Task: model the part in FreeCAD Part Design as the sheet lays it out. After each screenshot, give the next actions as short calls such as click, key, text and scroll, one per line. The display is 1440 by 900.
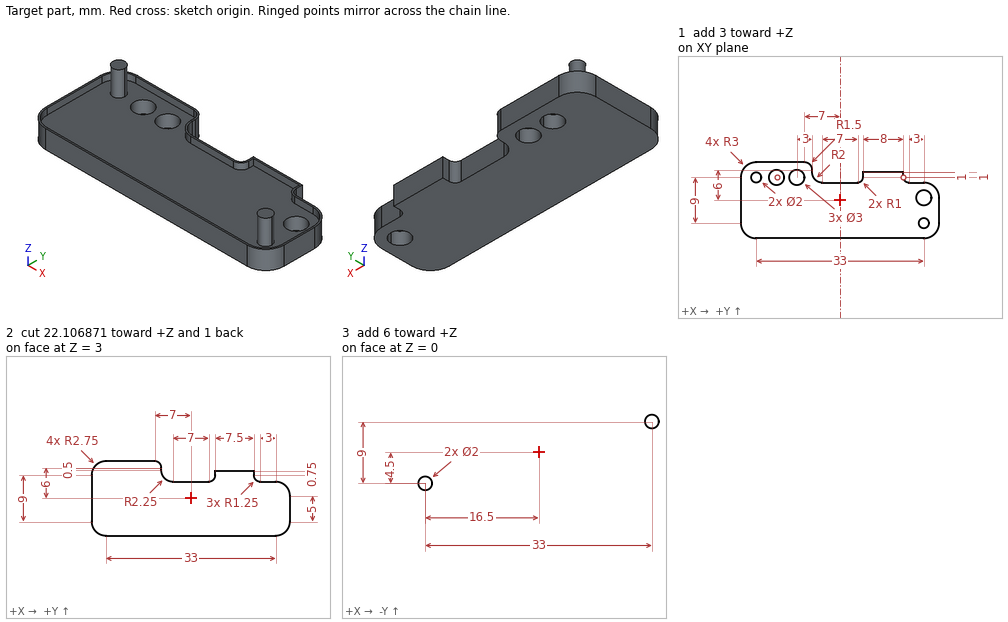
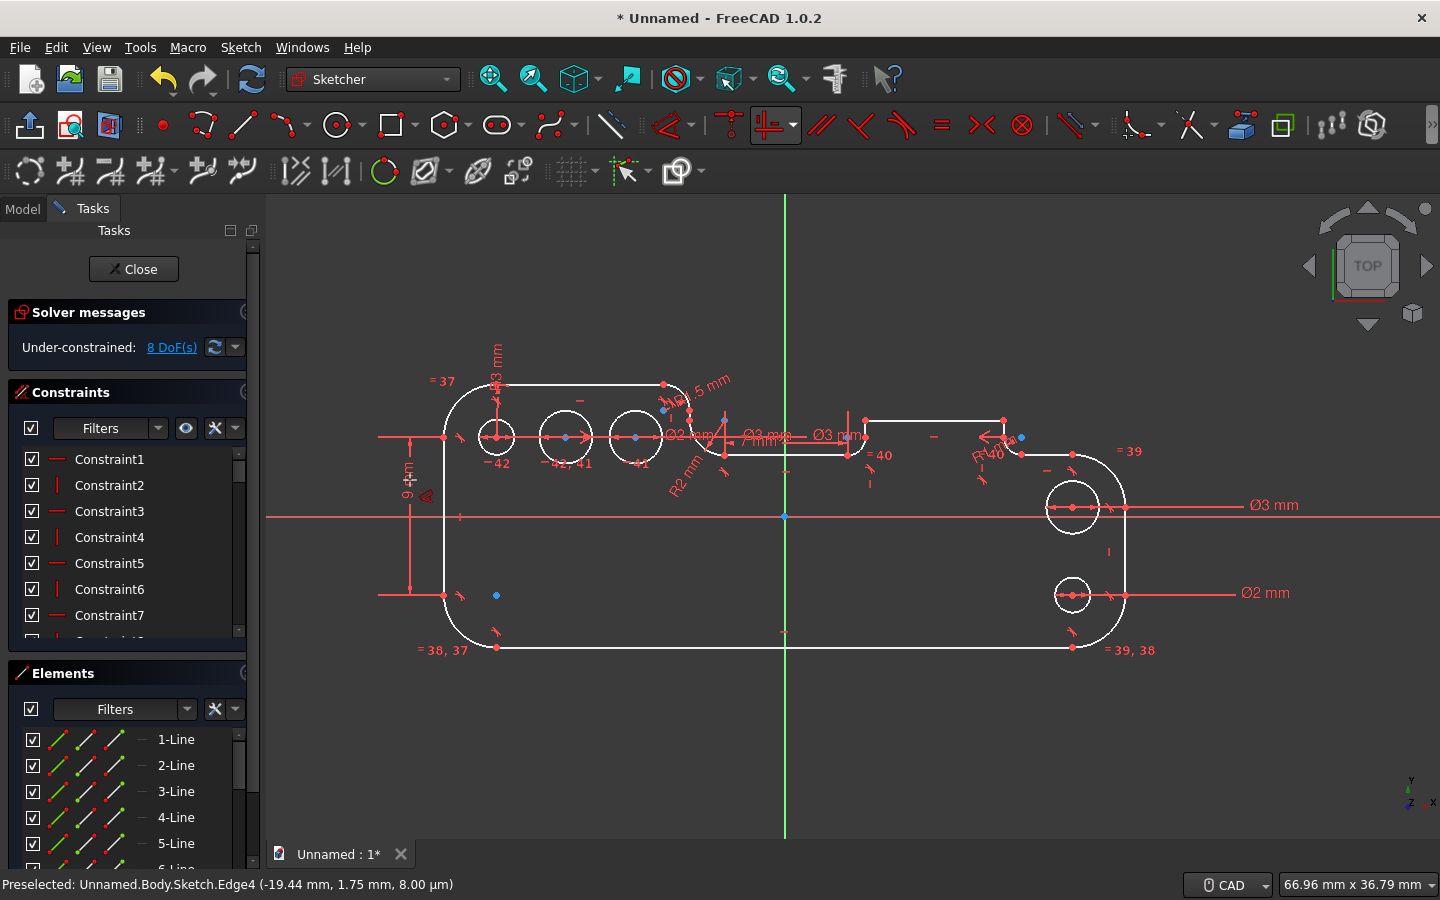
click(1057, 455)
click(1047, 421)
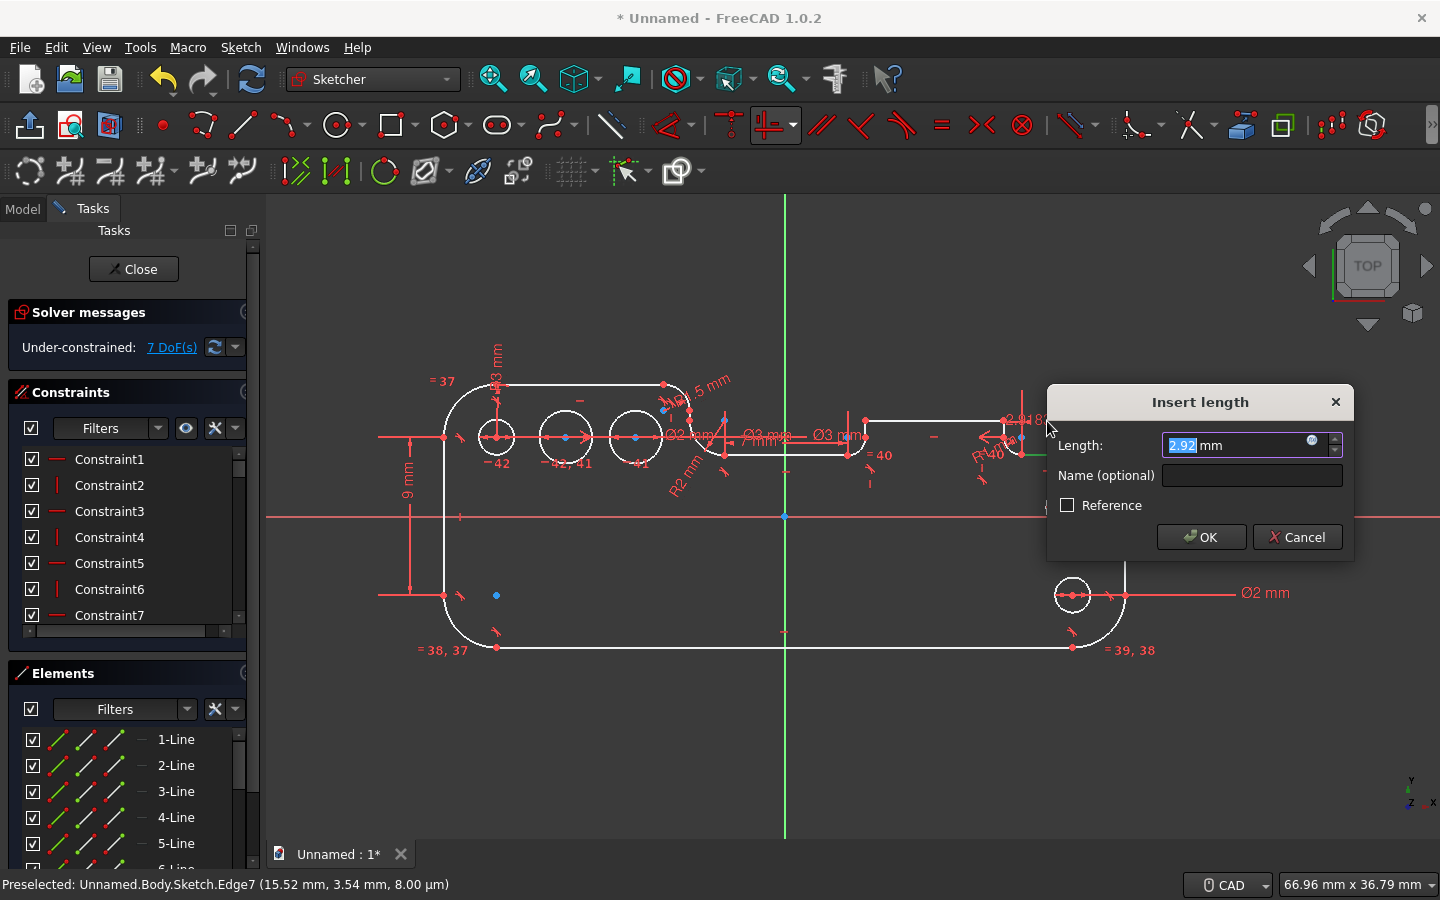
text(3)
key(Return)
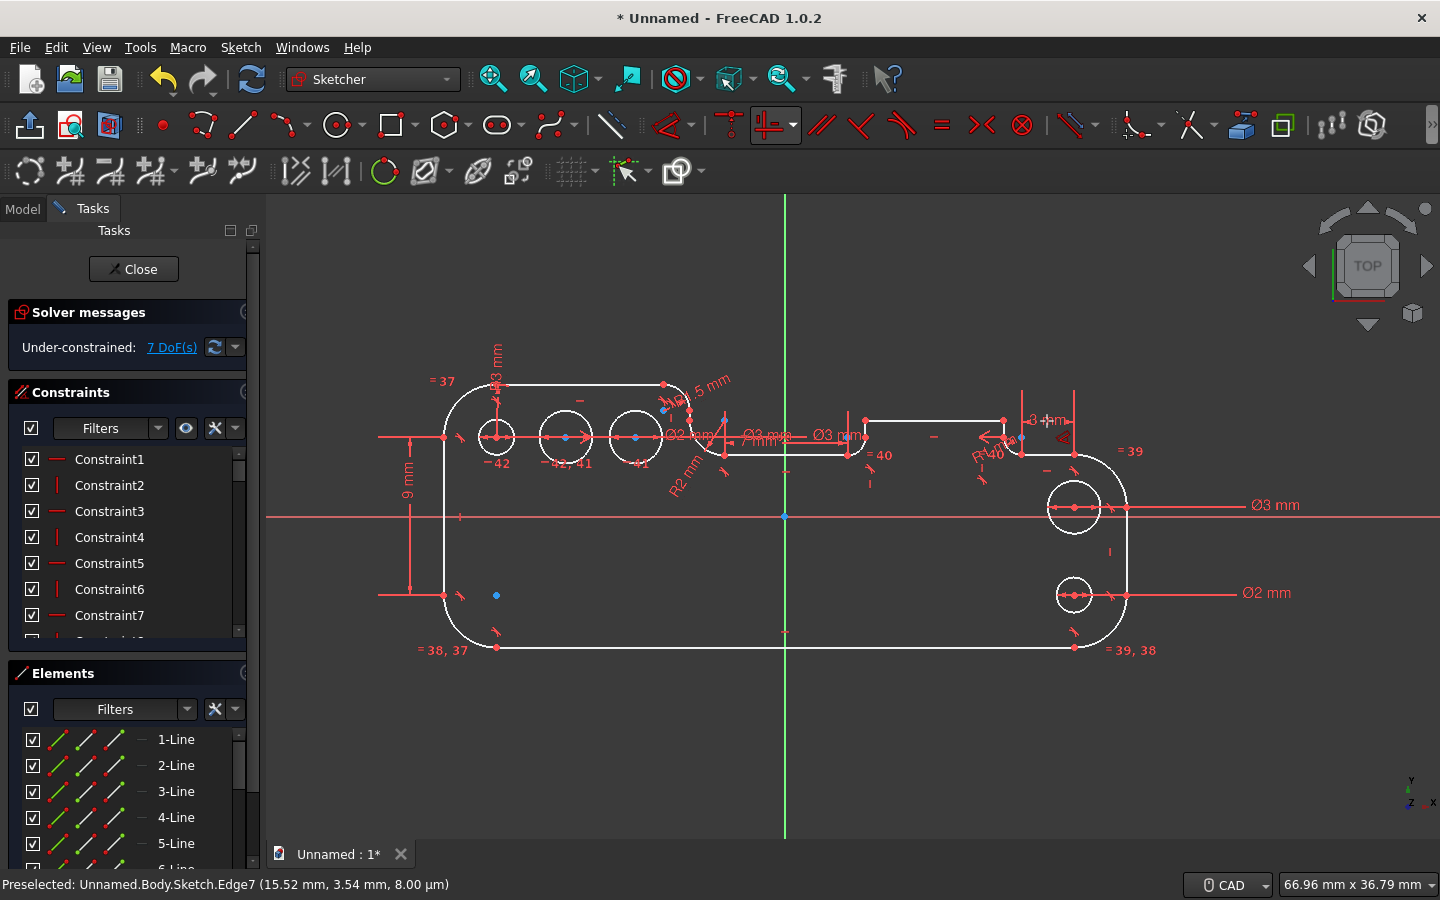
scroll(1004, 429, up, 5)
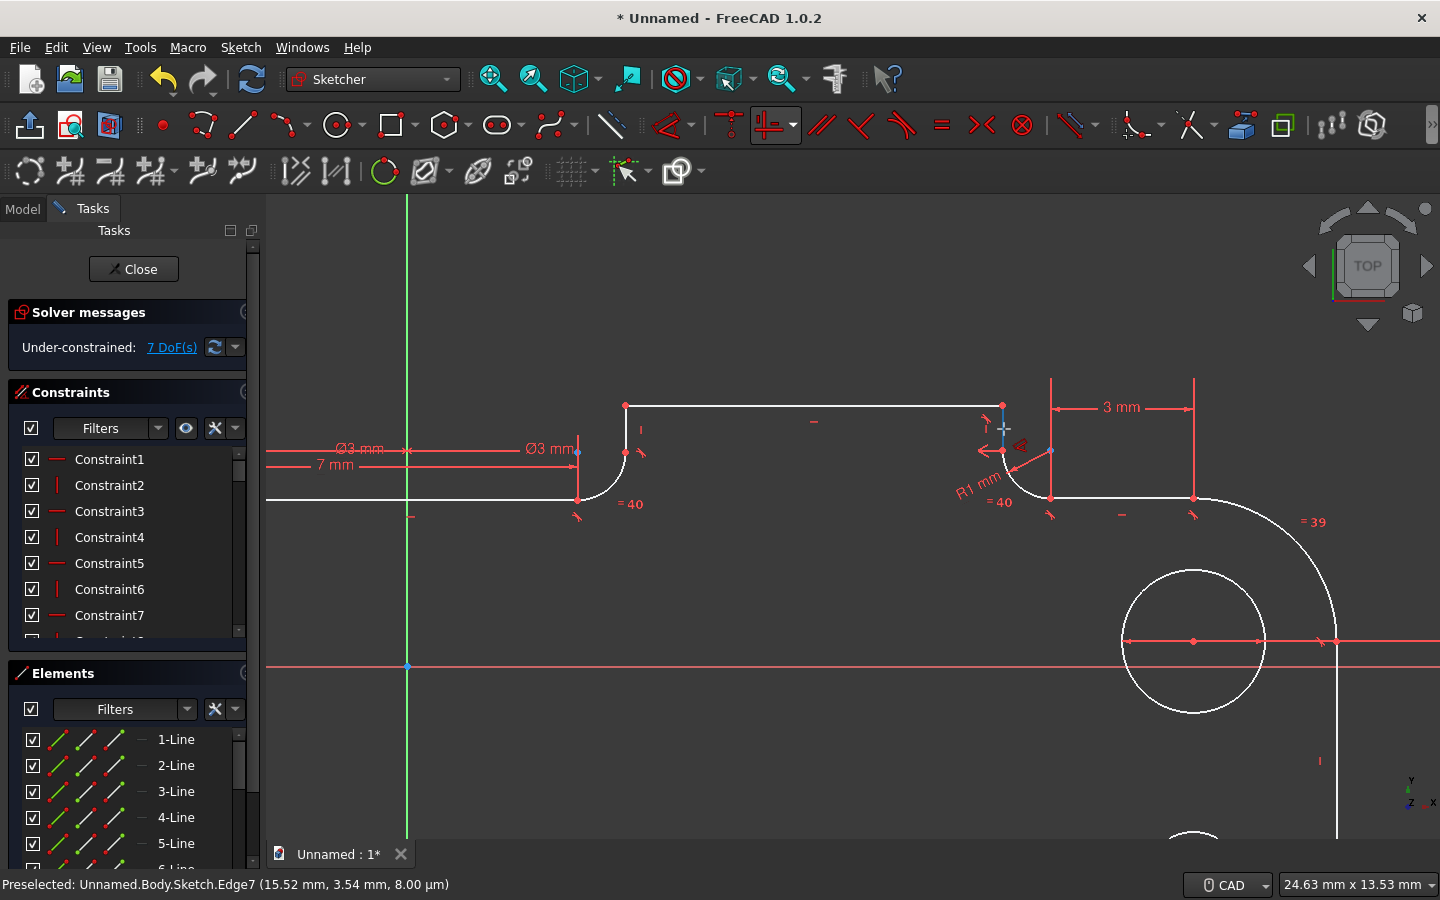
click(1003, 428)
click(1037, 428)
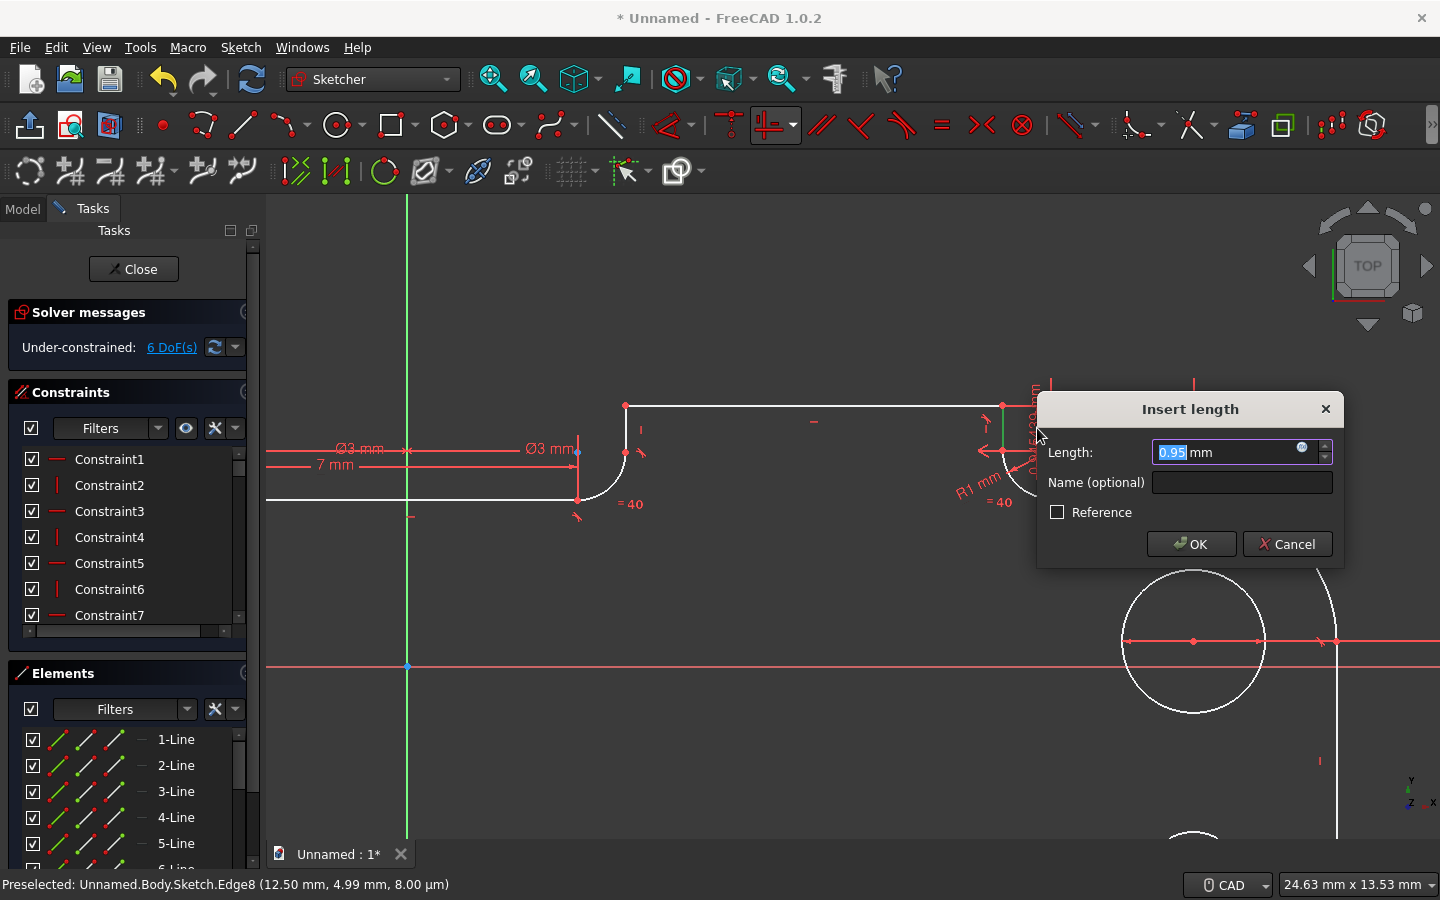
text(1)
key(Return)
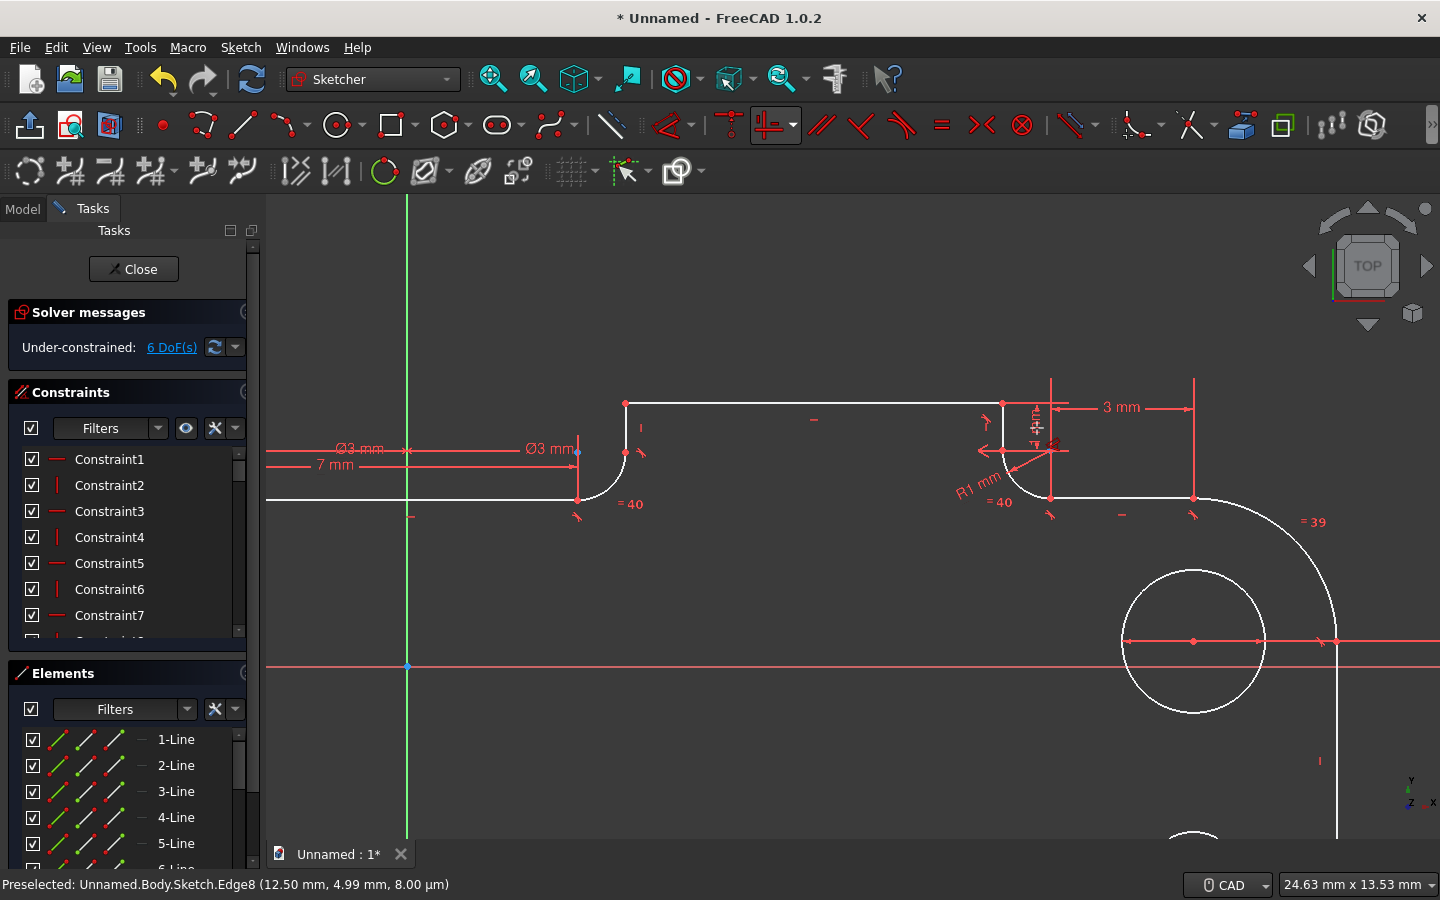
click(890, 403)
click(814, 369)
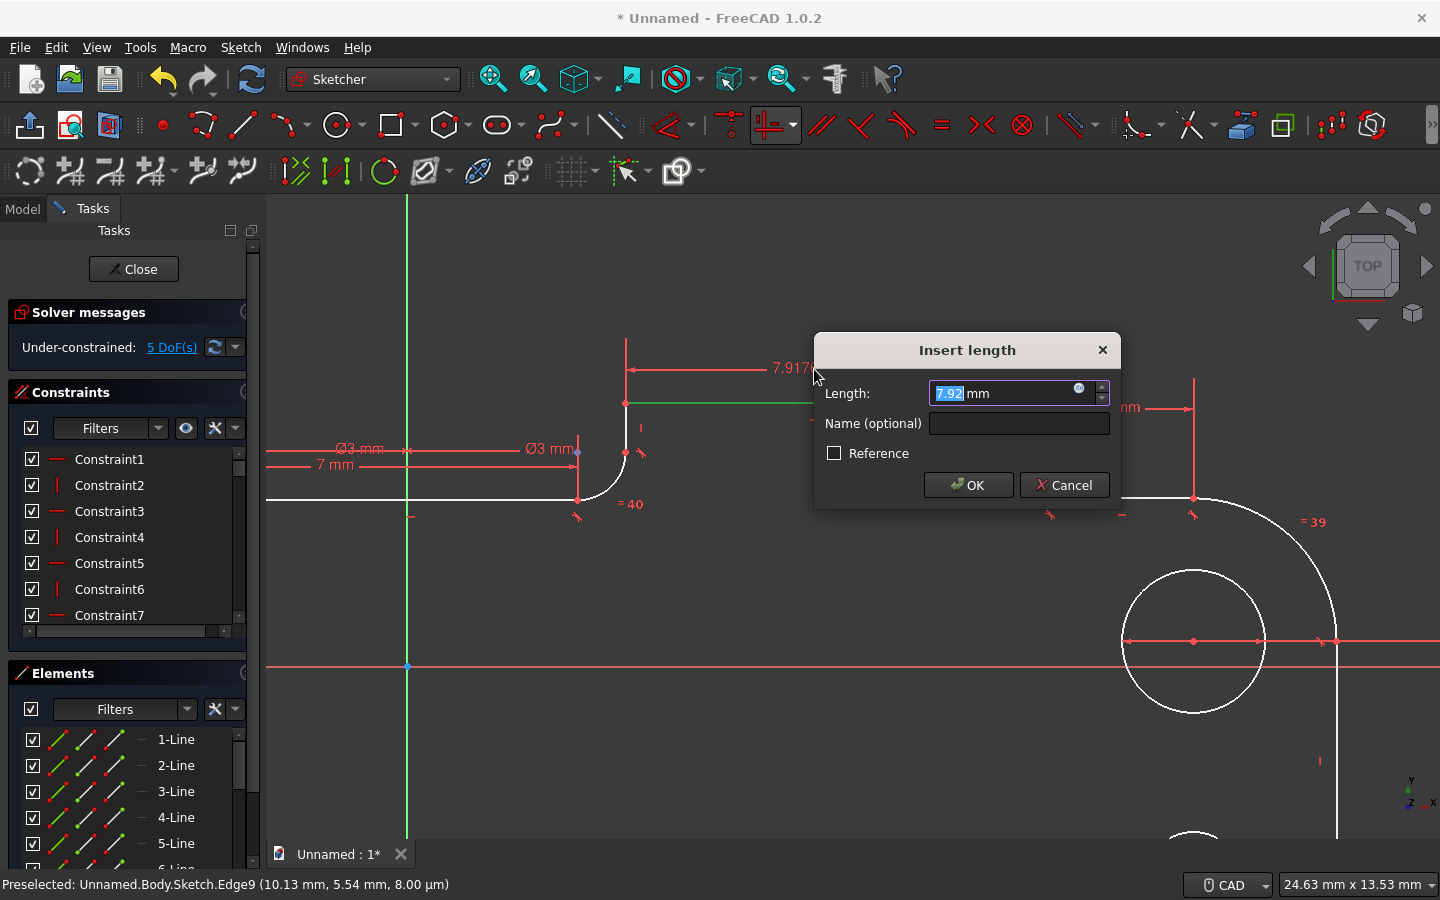
text(8)
key(Return)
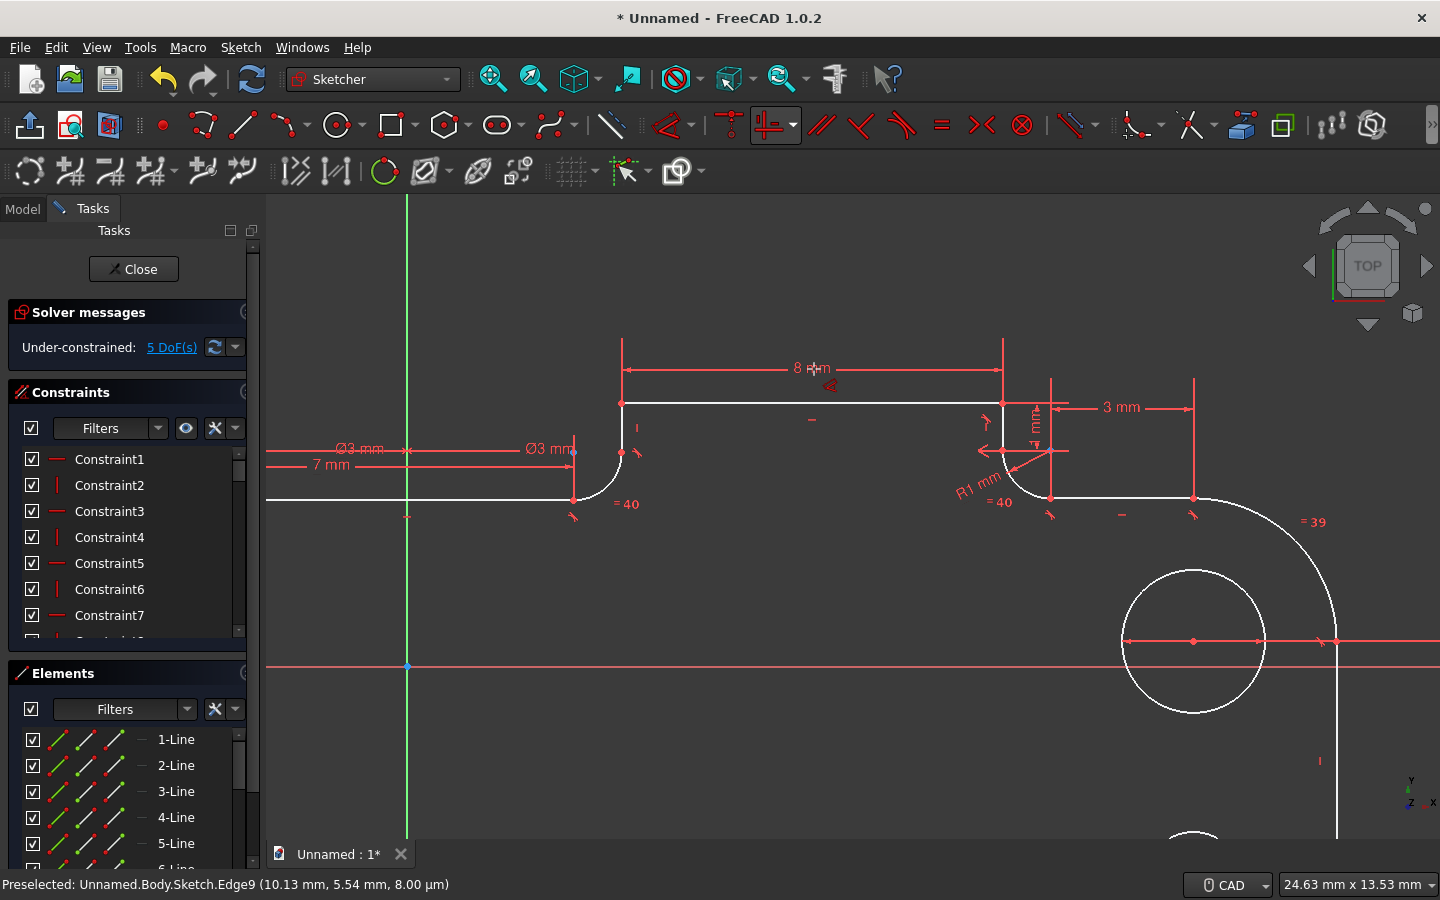
click(622, 418)
click(656, 428)